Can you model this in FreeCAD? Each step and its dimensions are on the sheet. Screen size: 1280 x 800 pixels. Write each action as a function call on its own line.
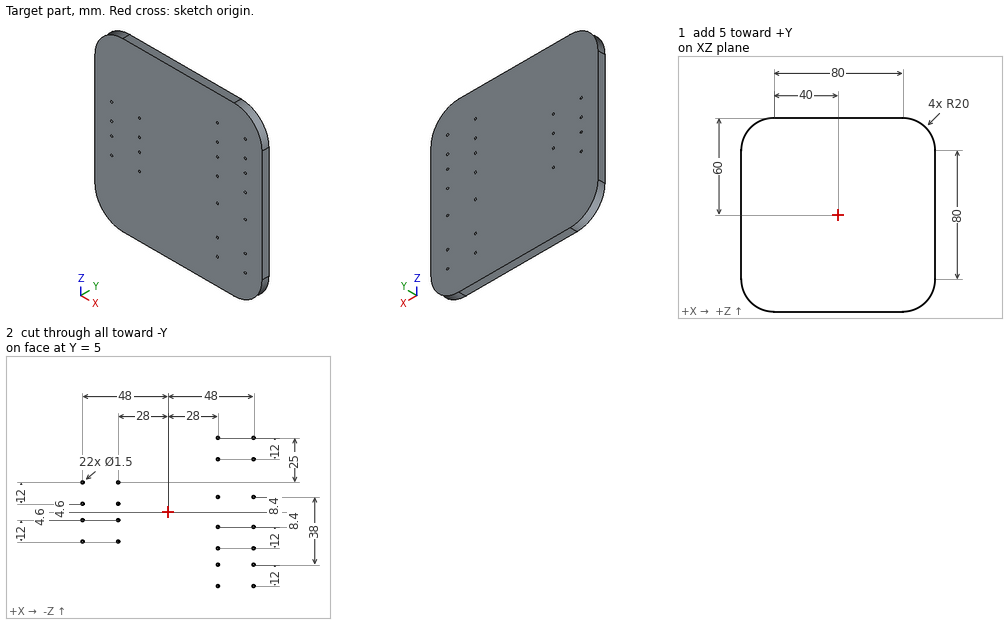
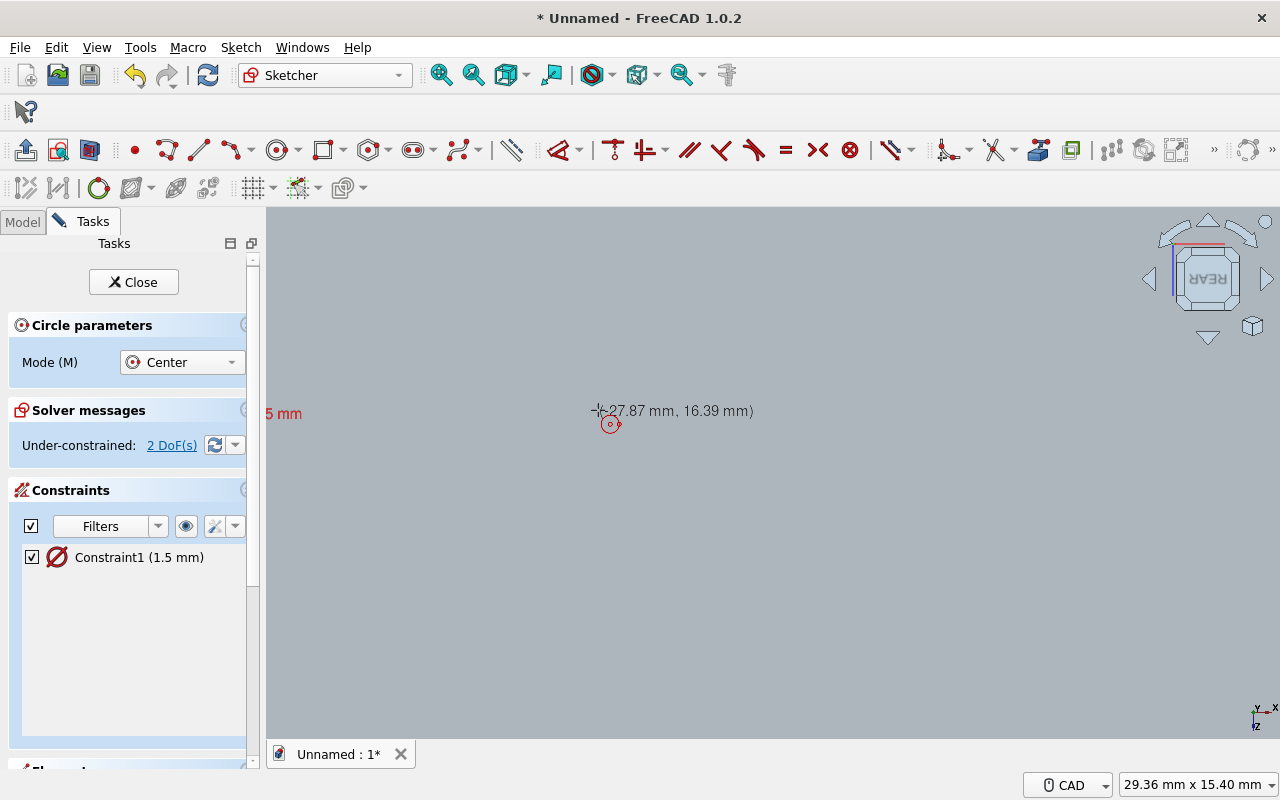
scroll(598, 410, down, 11)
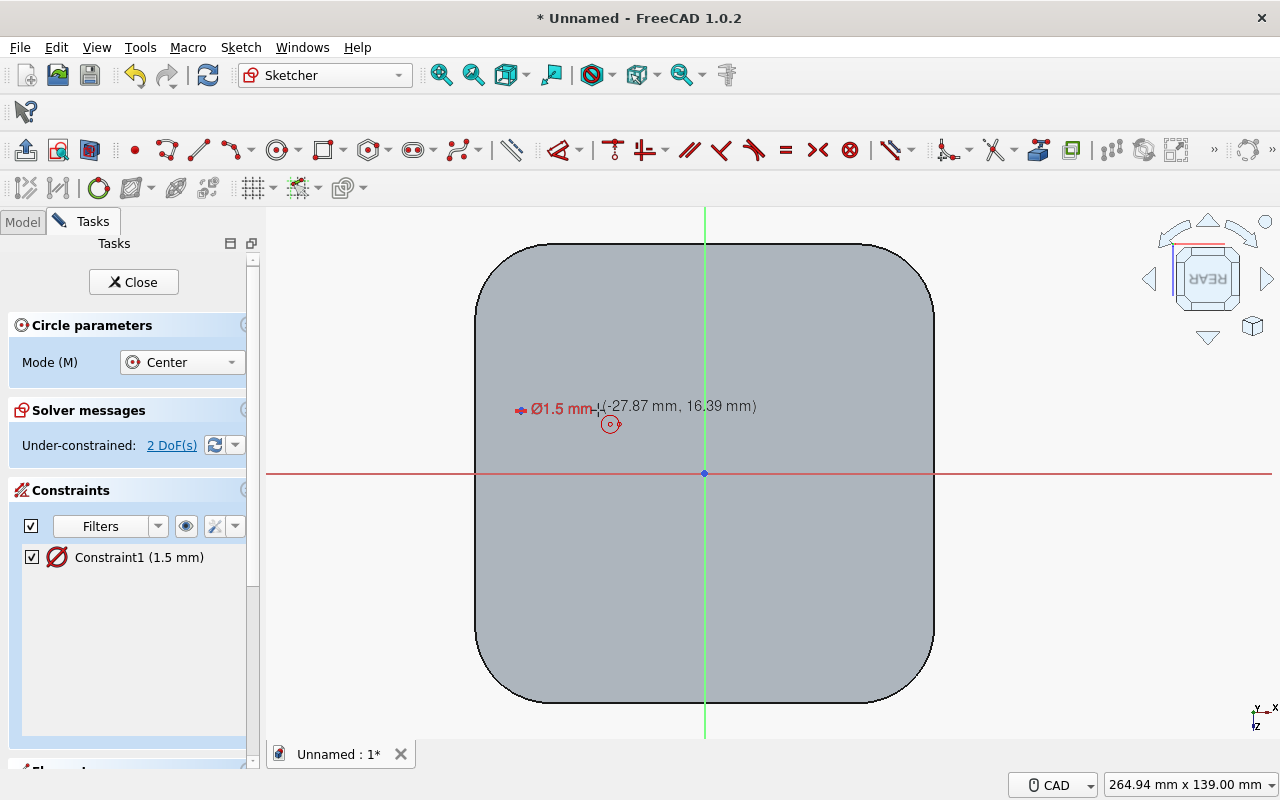
click(598, 410)
move(600, 408)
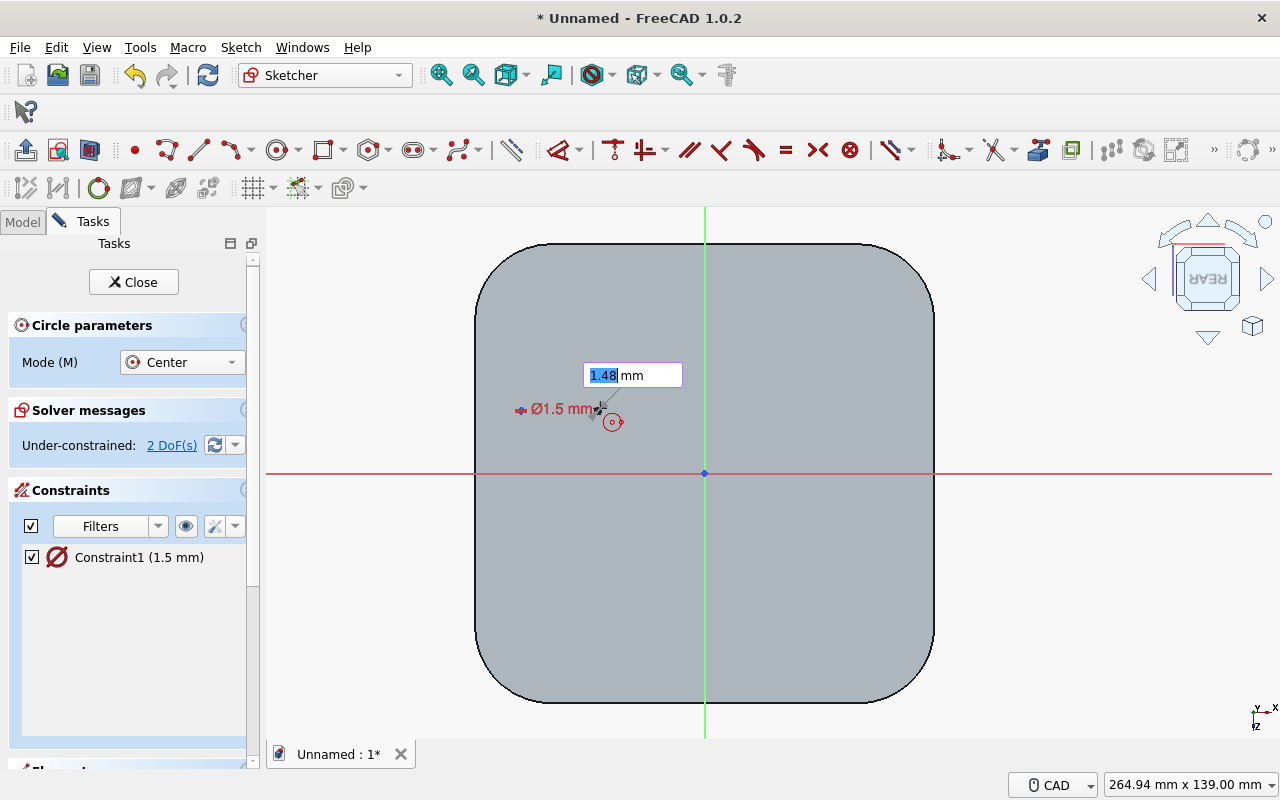
text(1.5)
key(Return)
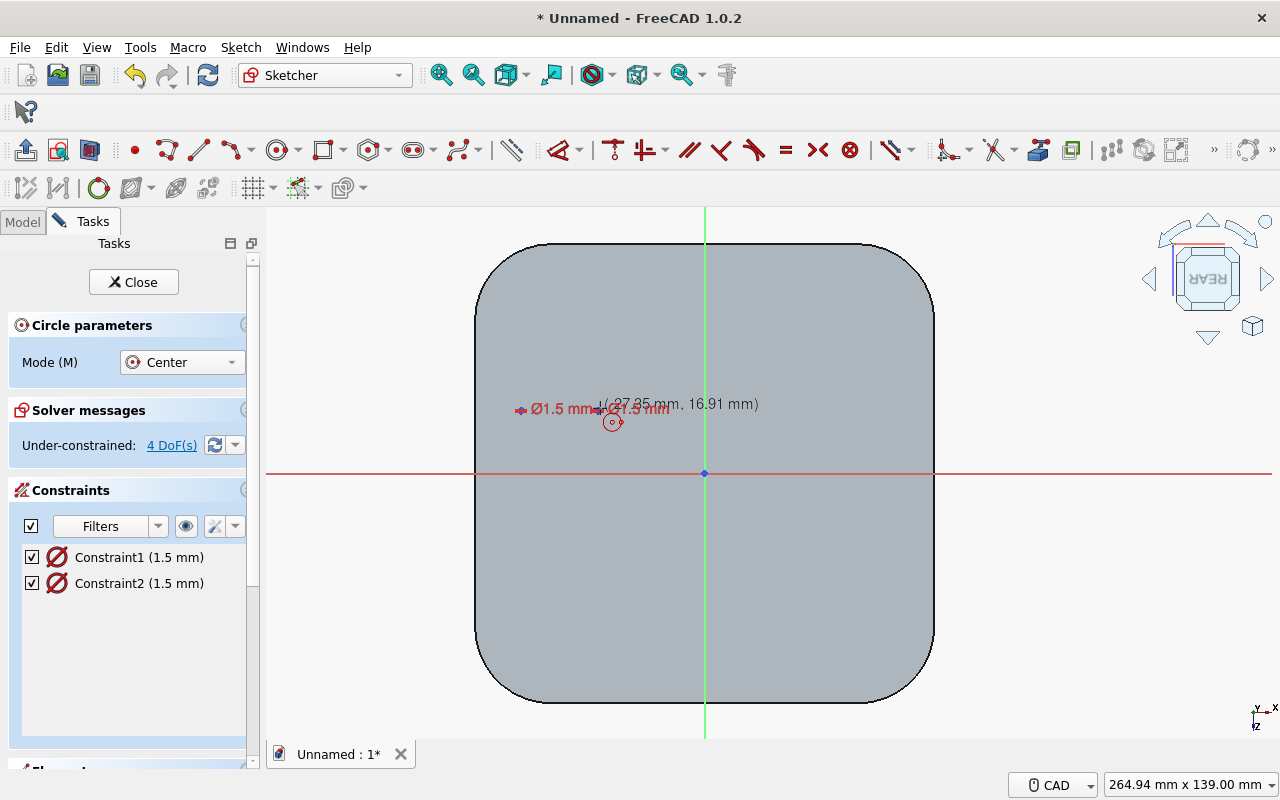
scroll(521, 456, up, 11)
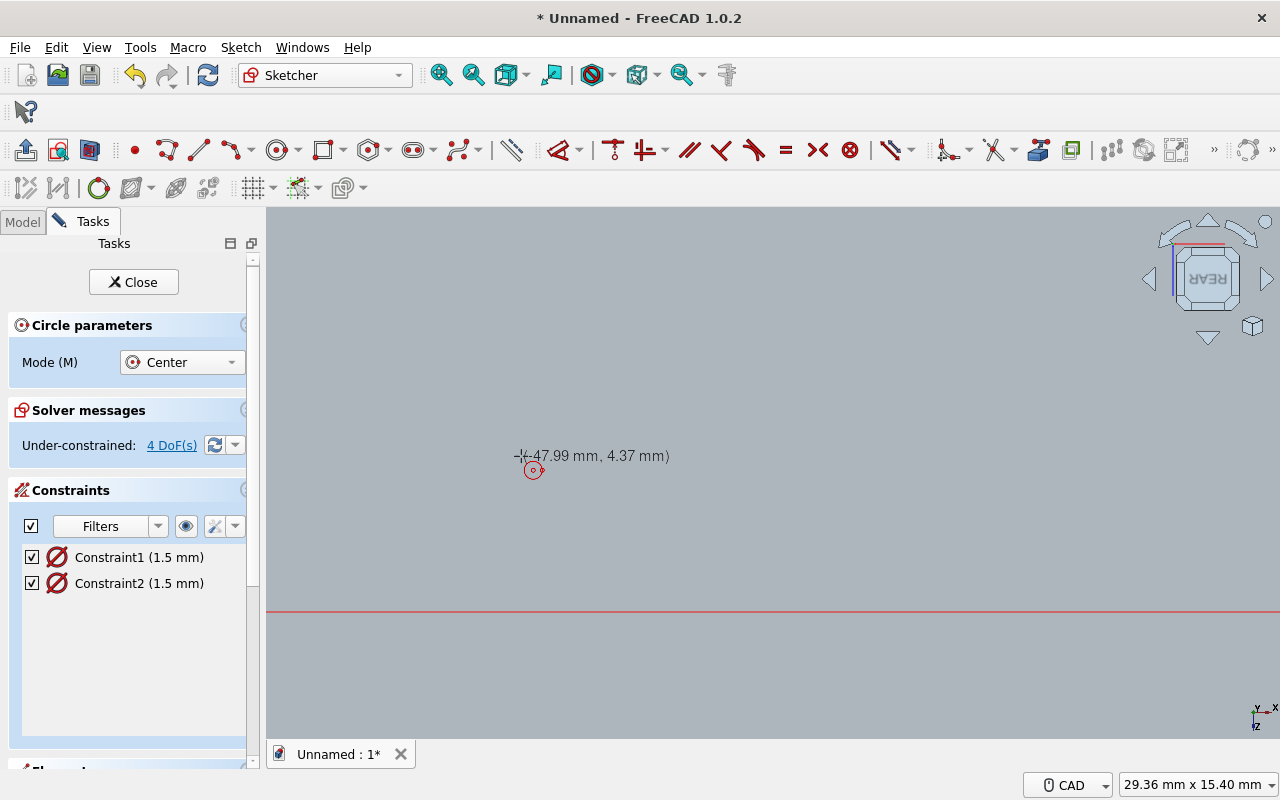
scroll(521, 456, down, 11)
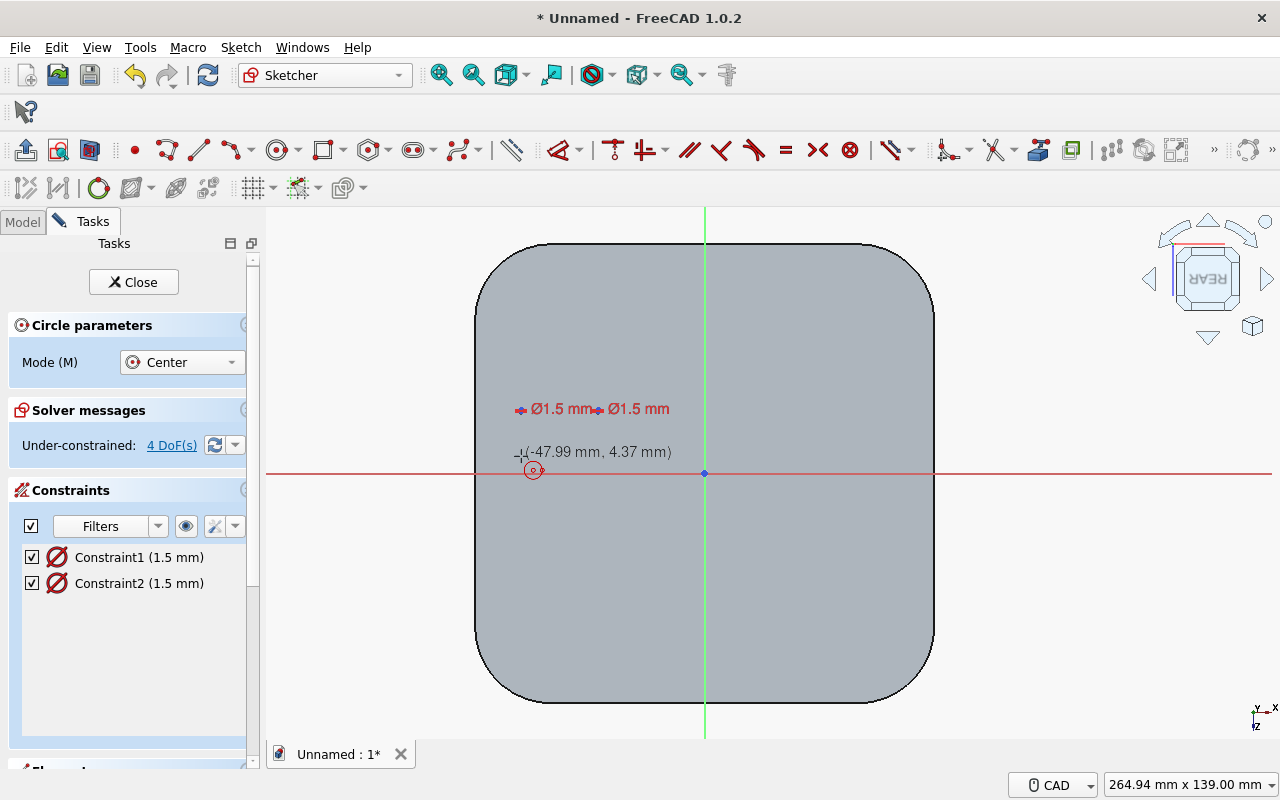
click(521, 456)
move(523, 454)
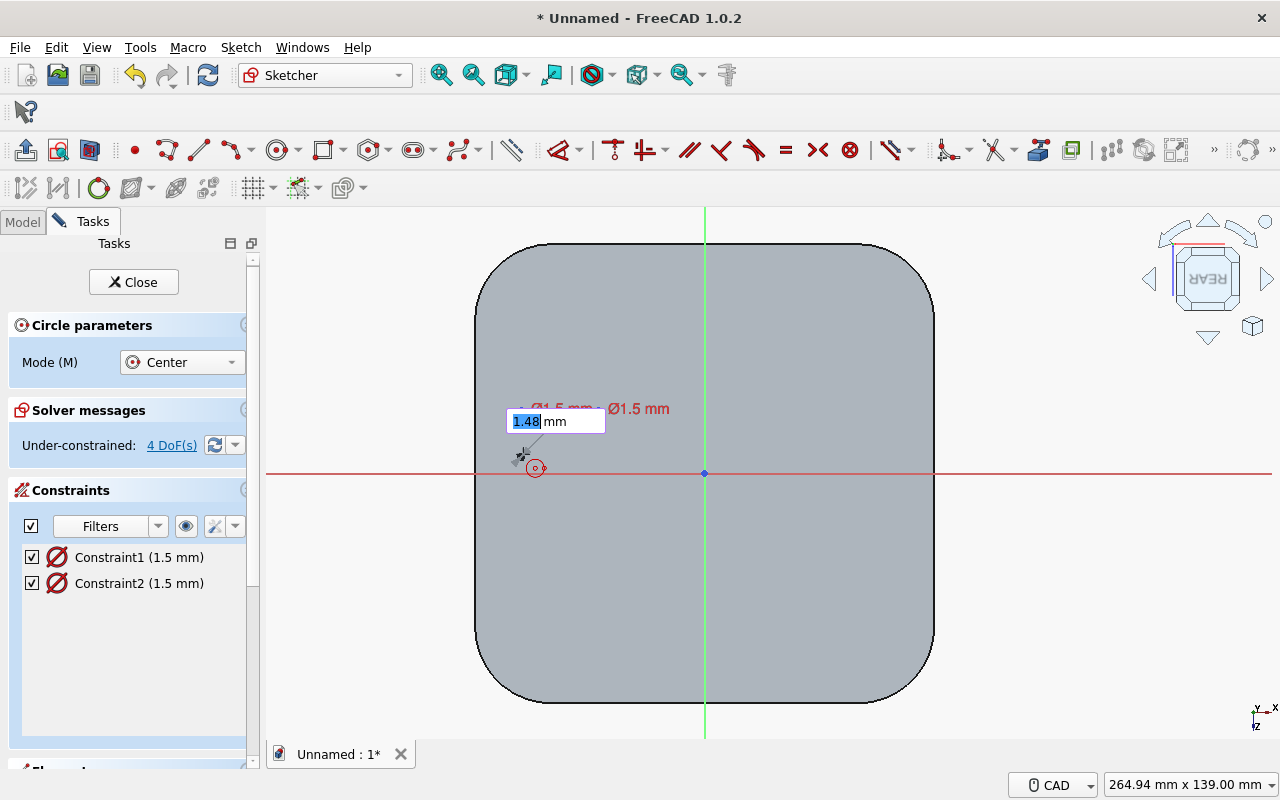
text(1.5)
key(Return)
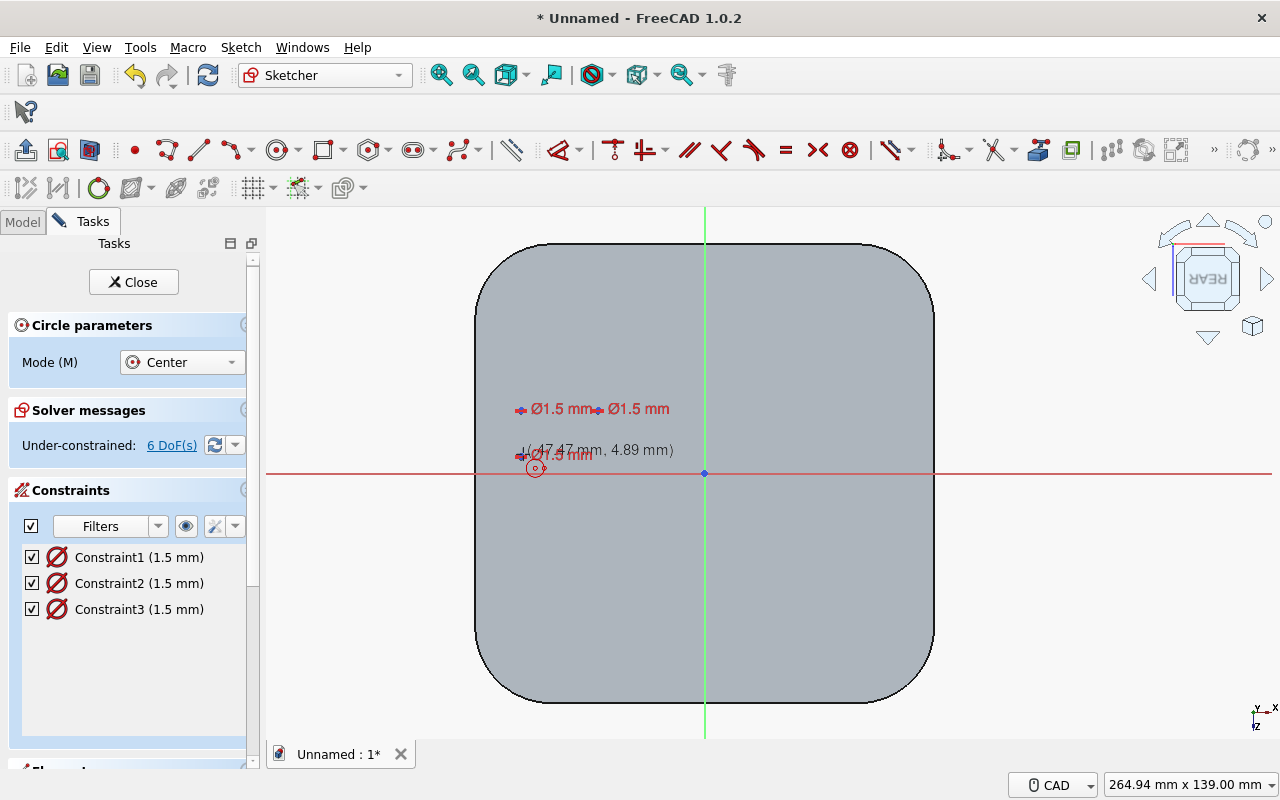
scroll(598, 456, up, 11)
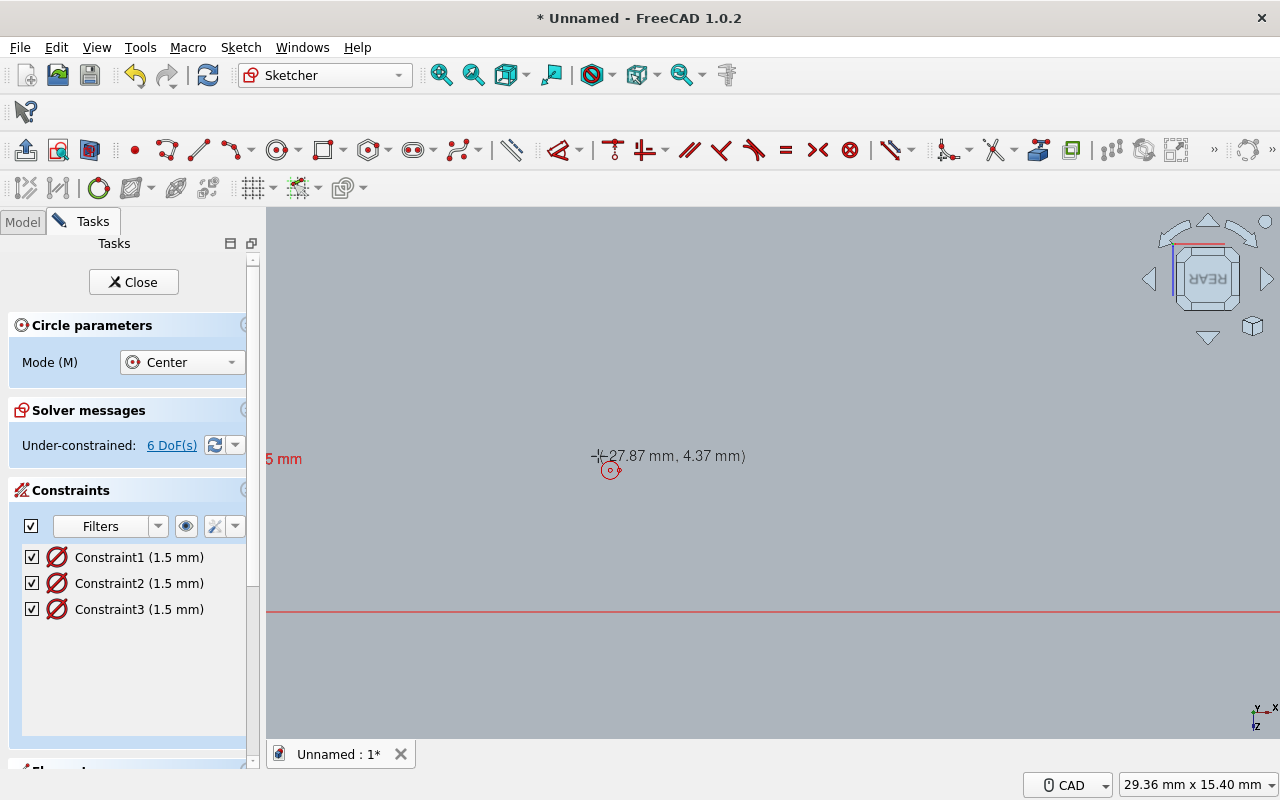
scroll(598, 456, down, 11)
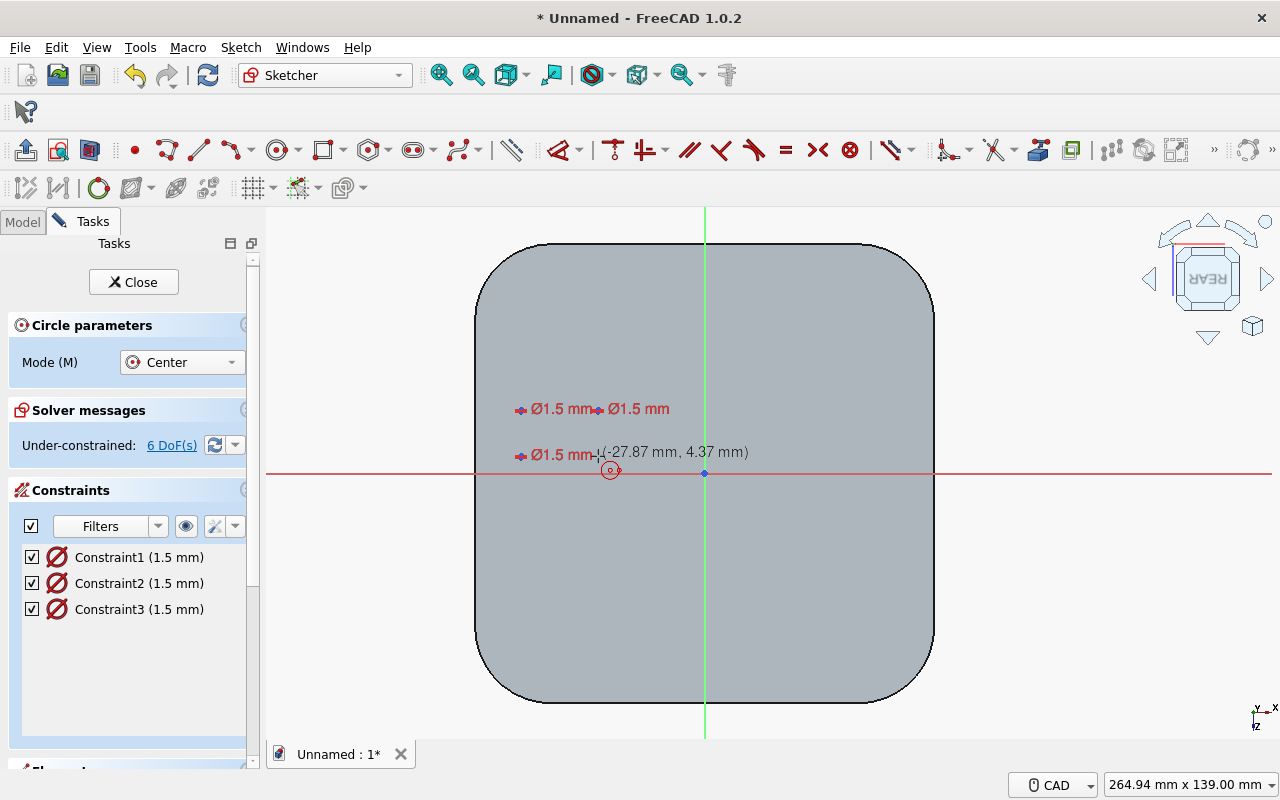
click(598, 456)
move(600, 454)